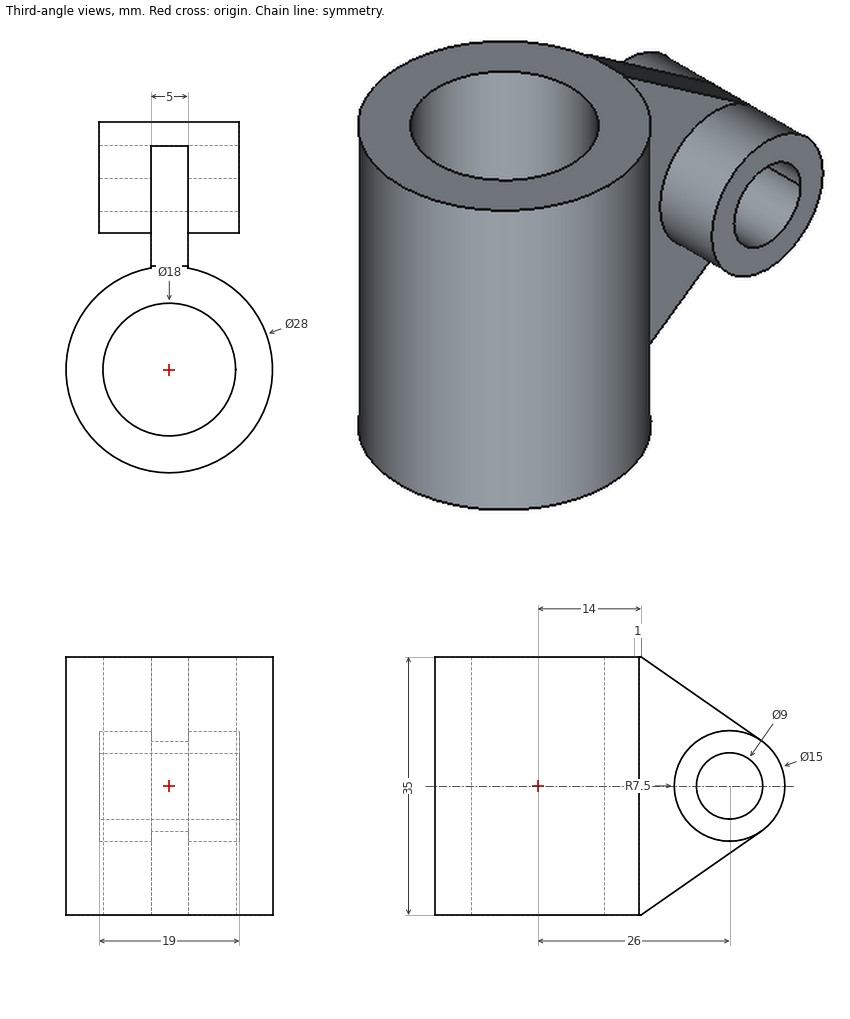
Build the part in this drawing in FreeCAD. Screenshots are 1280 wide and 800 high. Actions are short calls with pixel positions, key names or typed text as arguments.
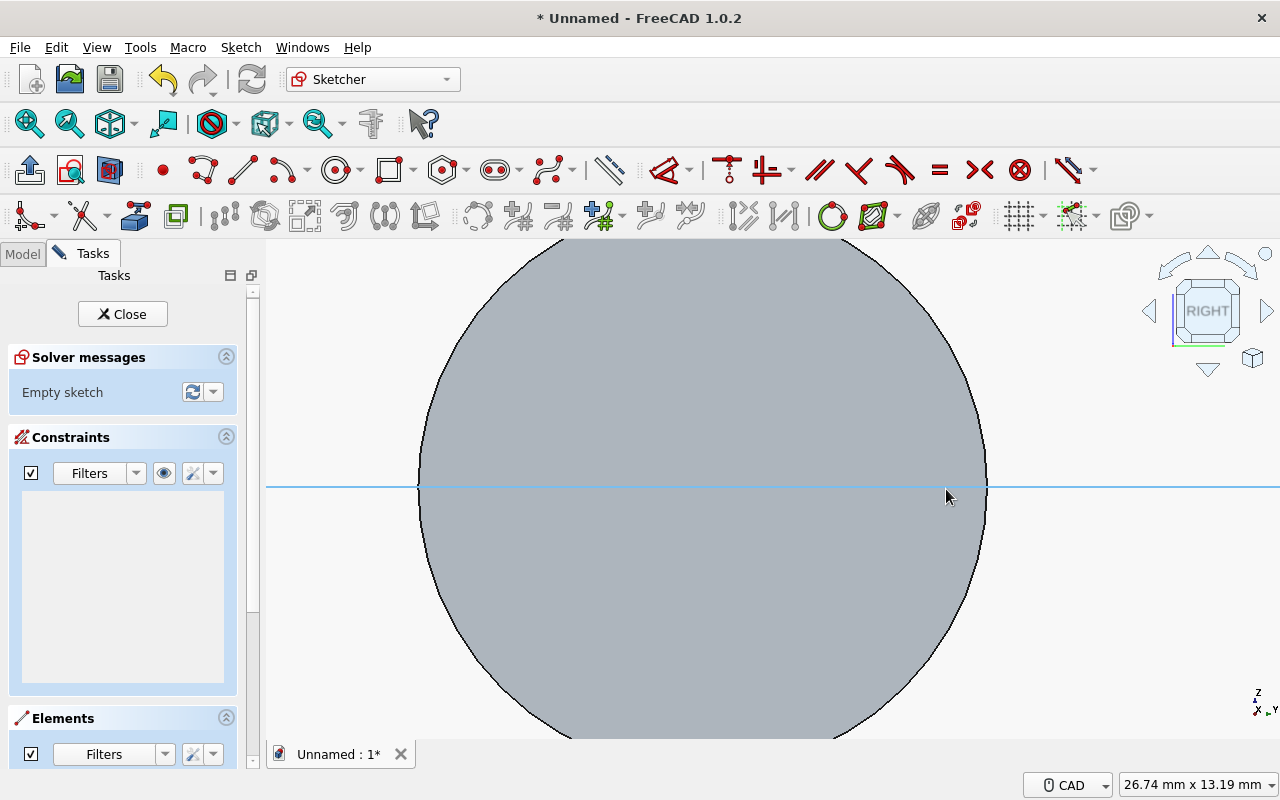
click(336, 170)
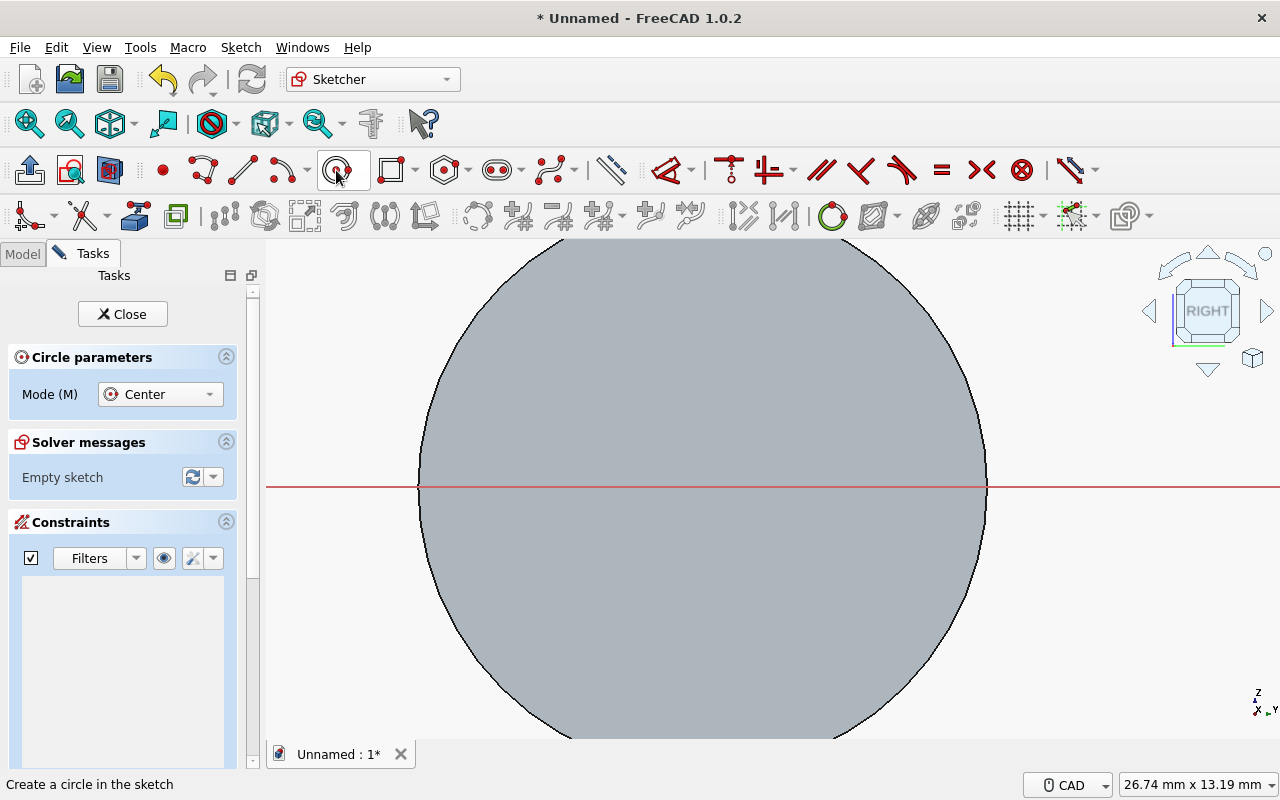
click(703, 487)
click(823, 366)
key(Escape)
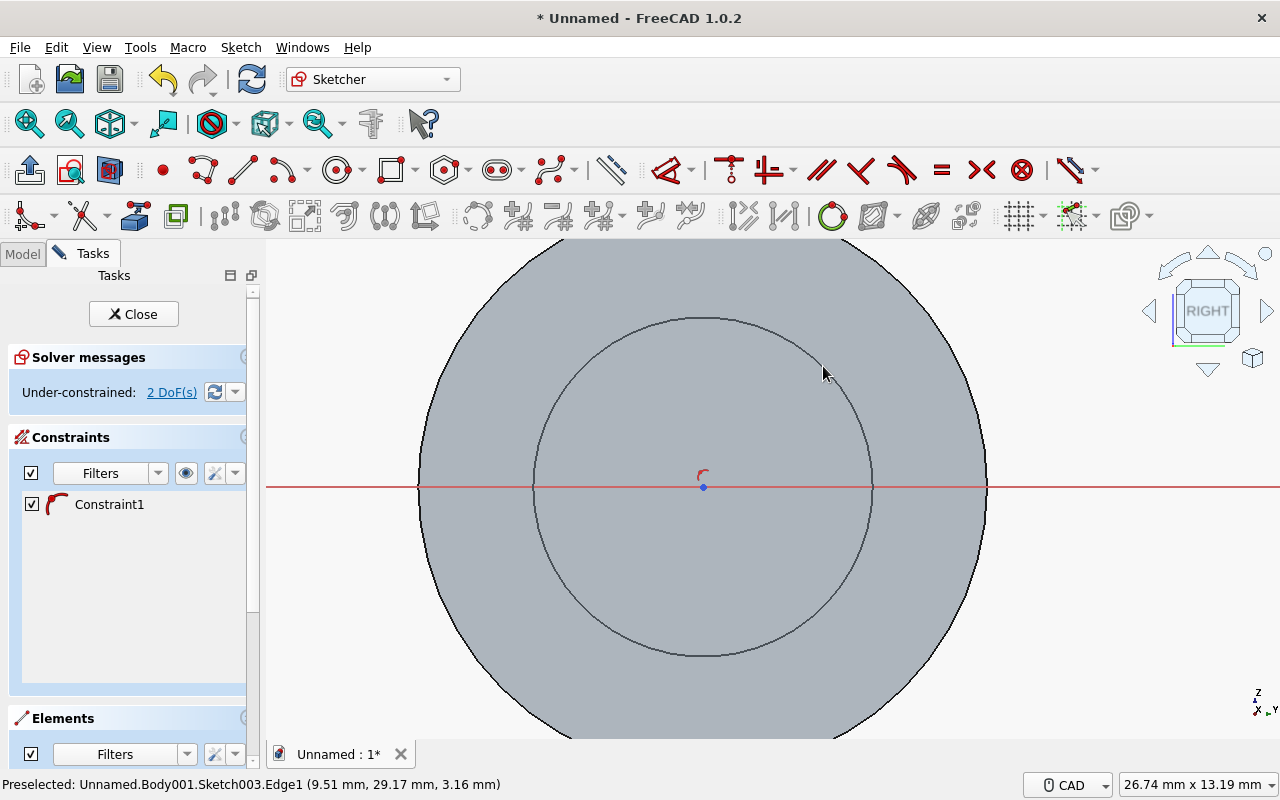
key(d)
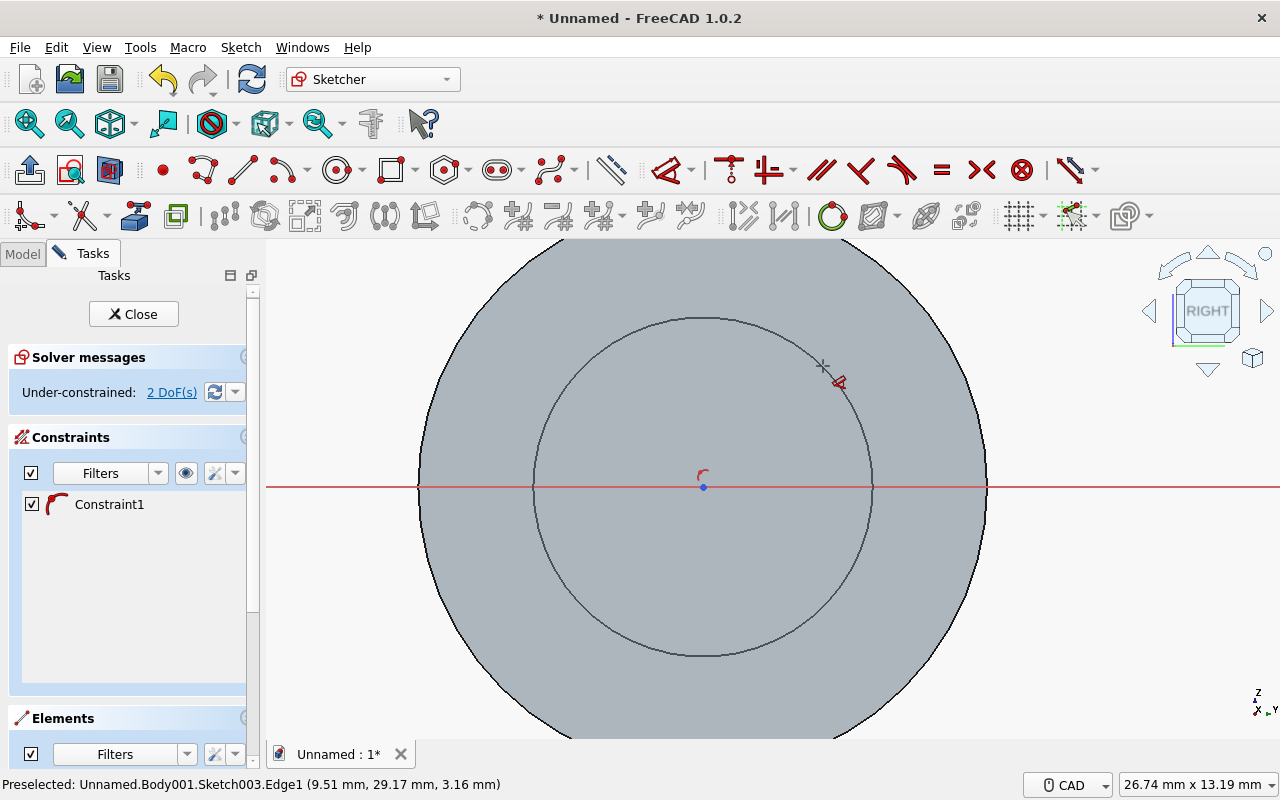
click(823, 367)
click(846, 344)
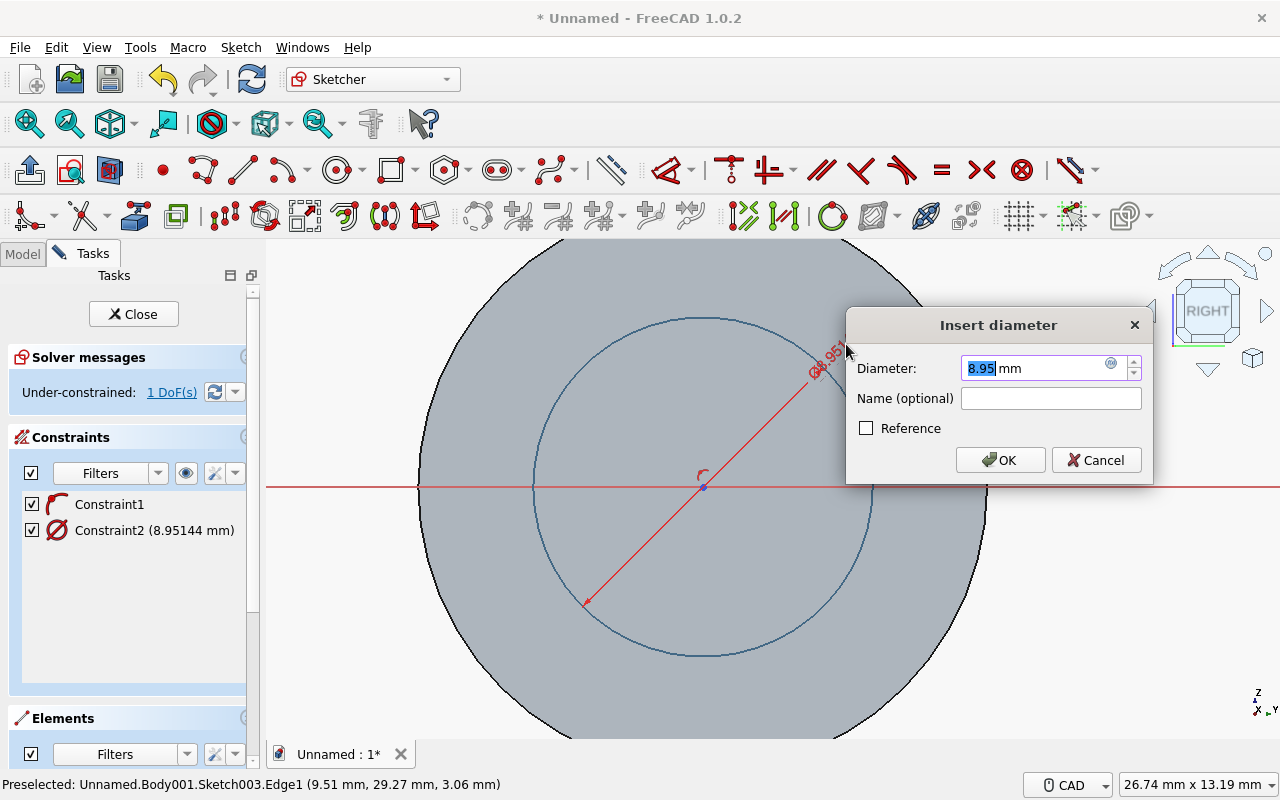
text(9)
key(Return)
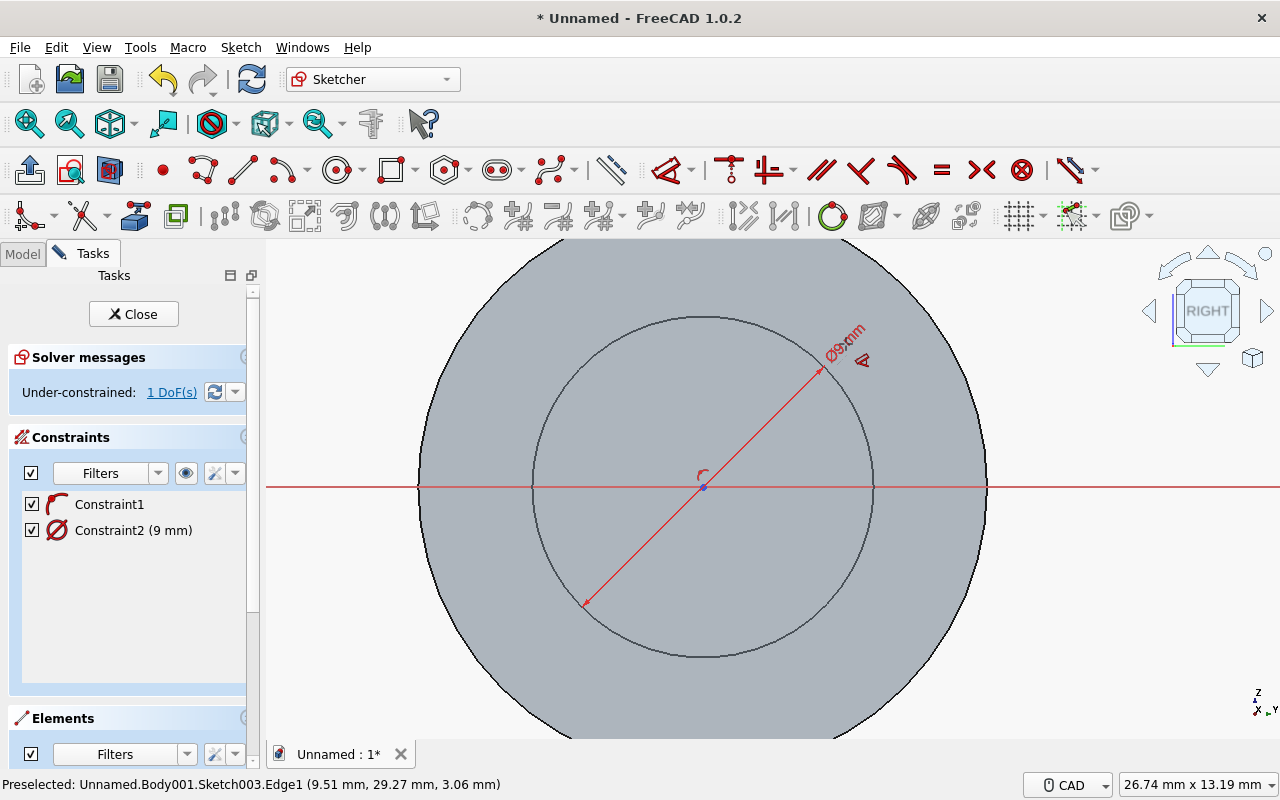
click(703, 487)
click(498, 521)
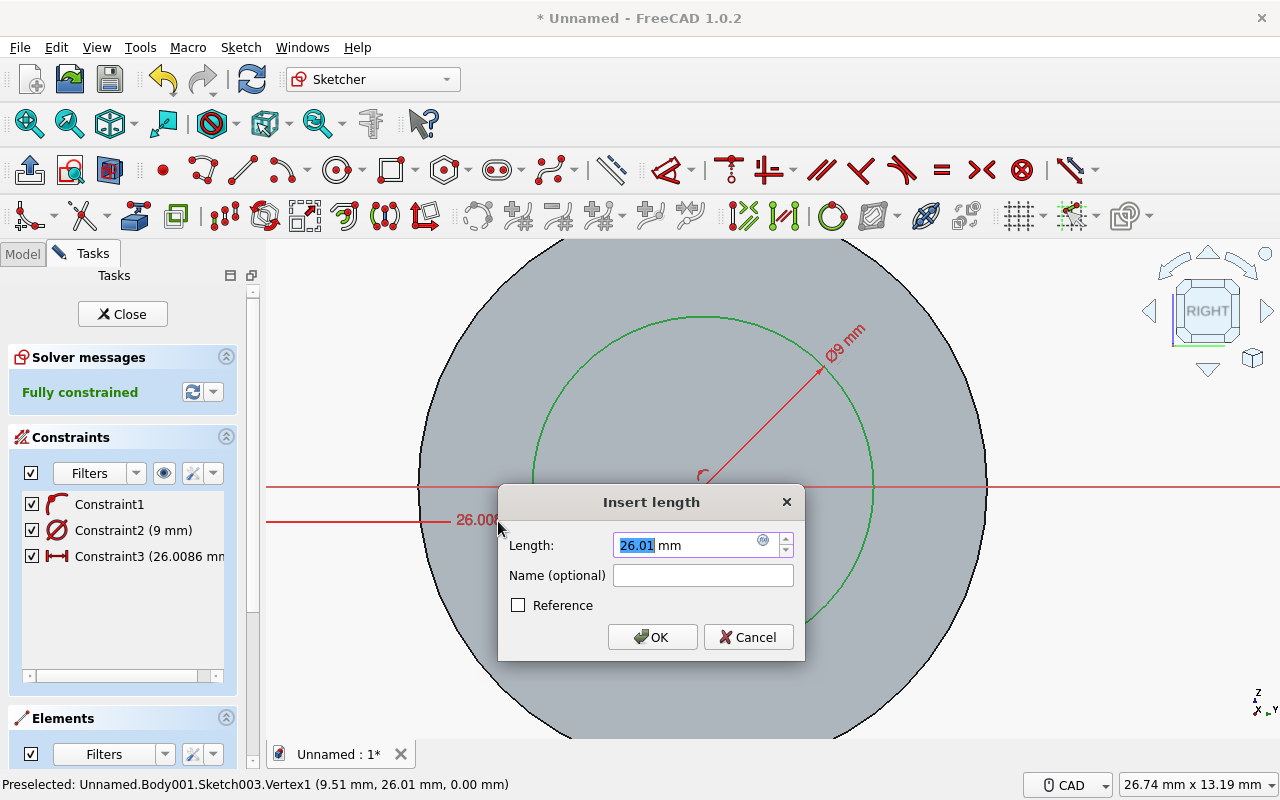
text(26)
key(Return)
key(Escape)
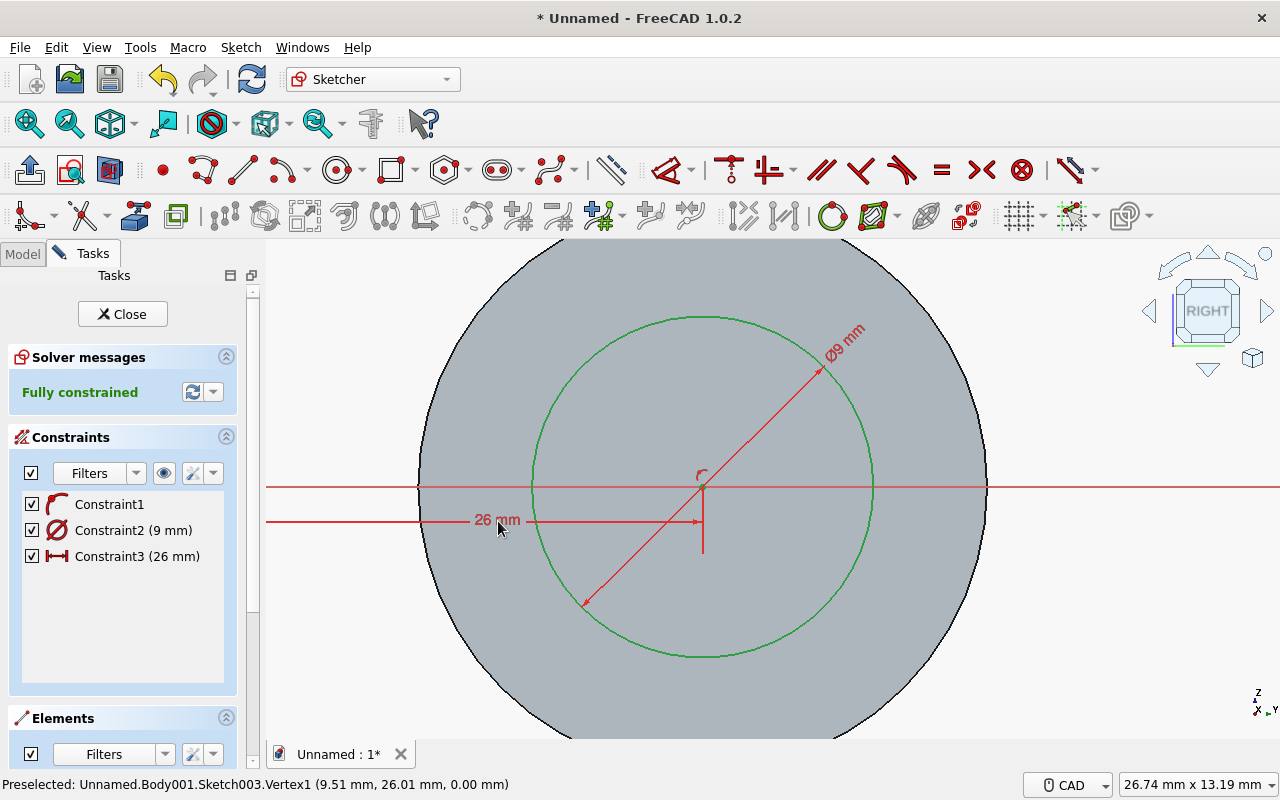
click(123, 314)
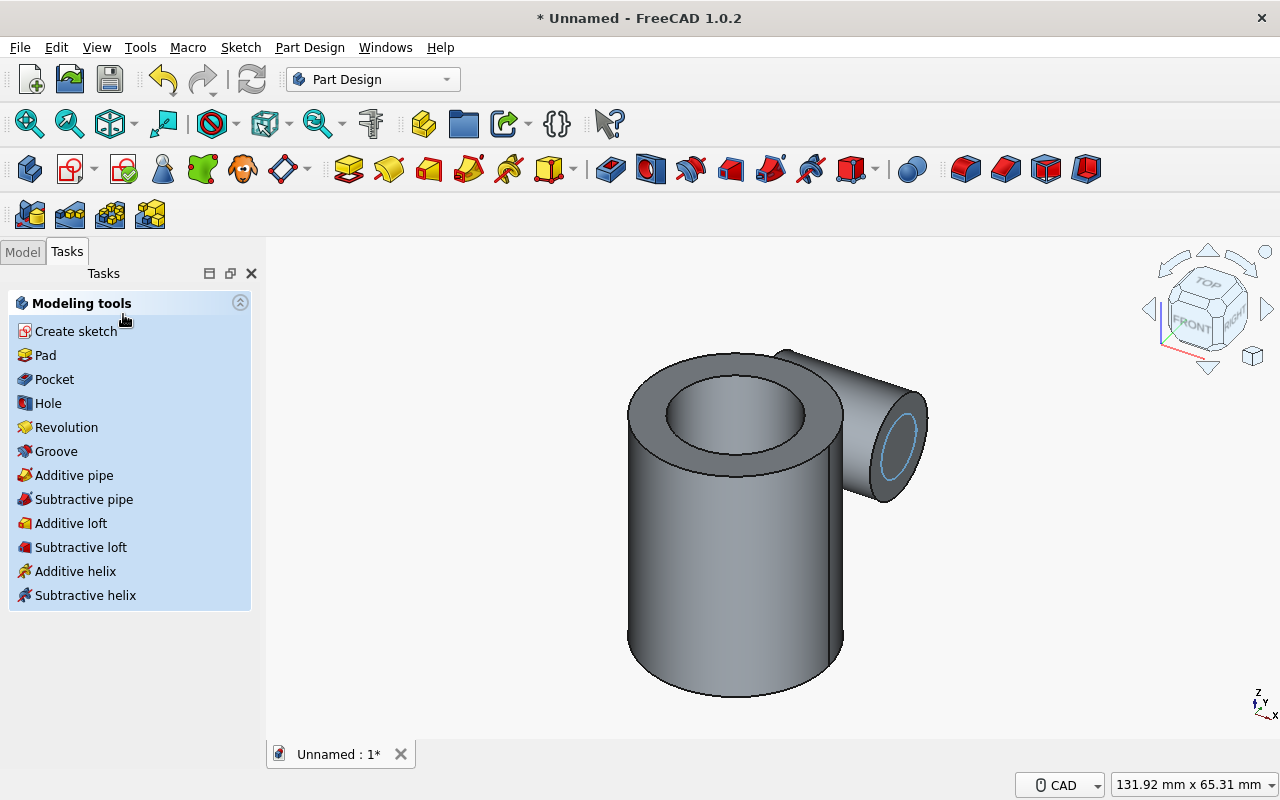
click(612, 170)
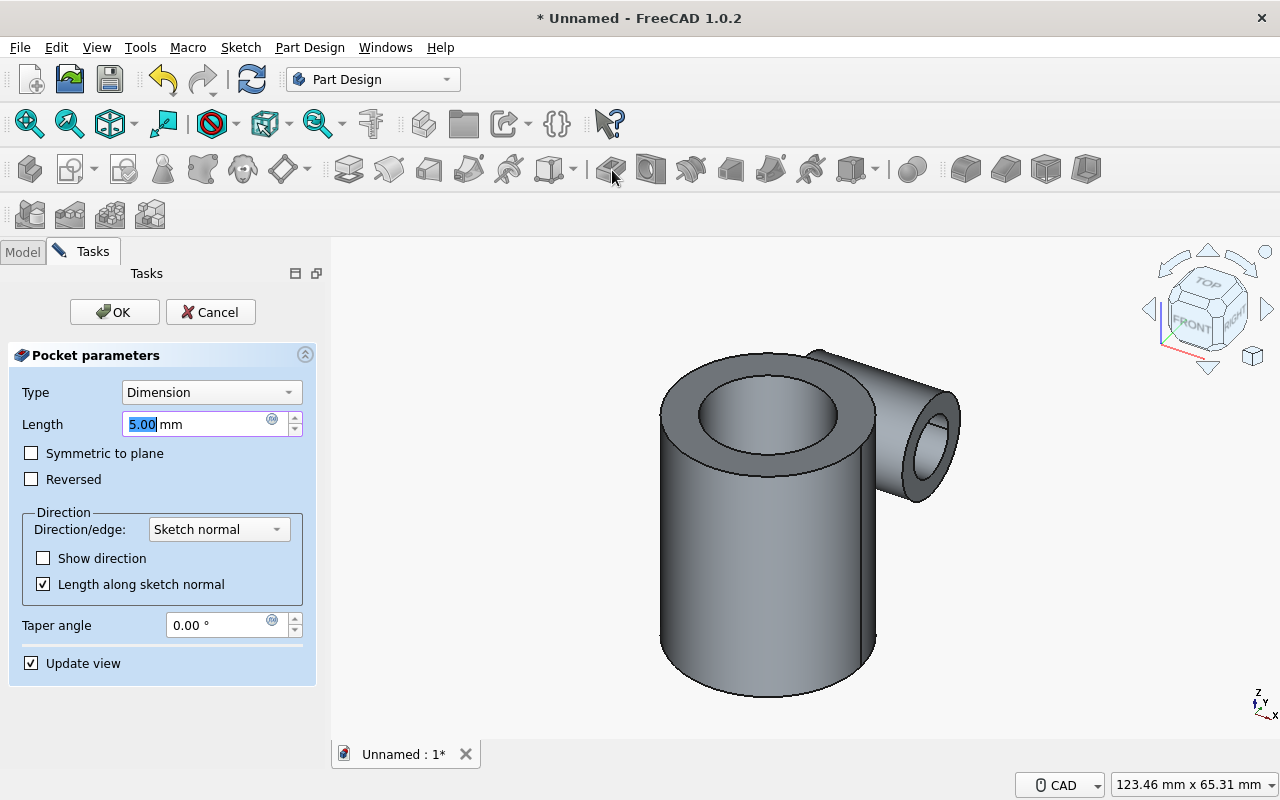
click(212, 392)